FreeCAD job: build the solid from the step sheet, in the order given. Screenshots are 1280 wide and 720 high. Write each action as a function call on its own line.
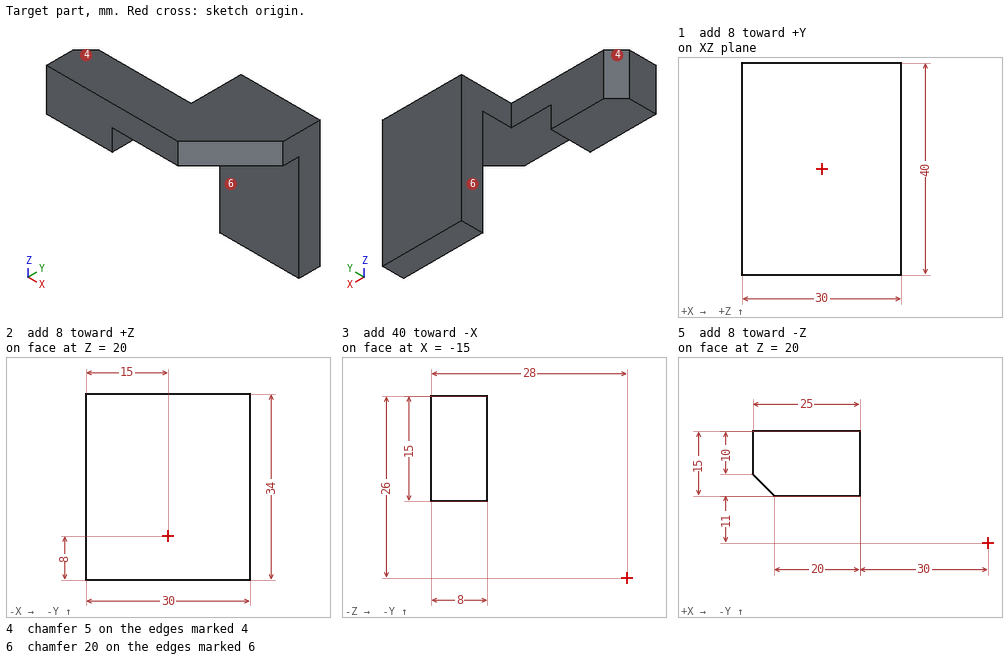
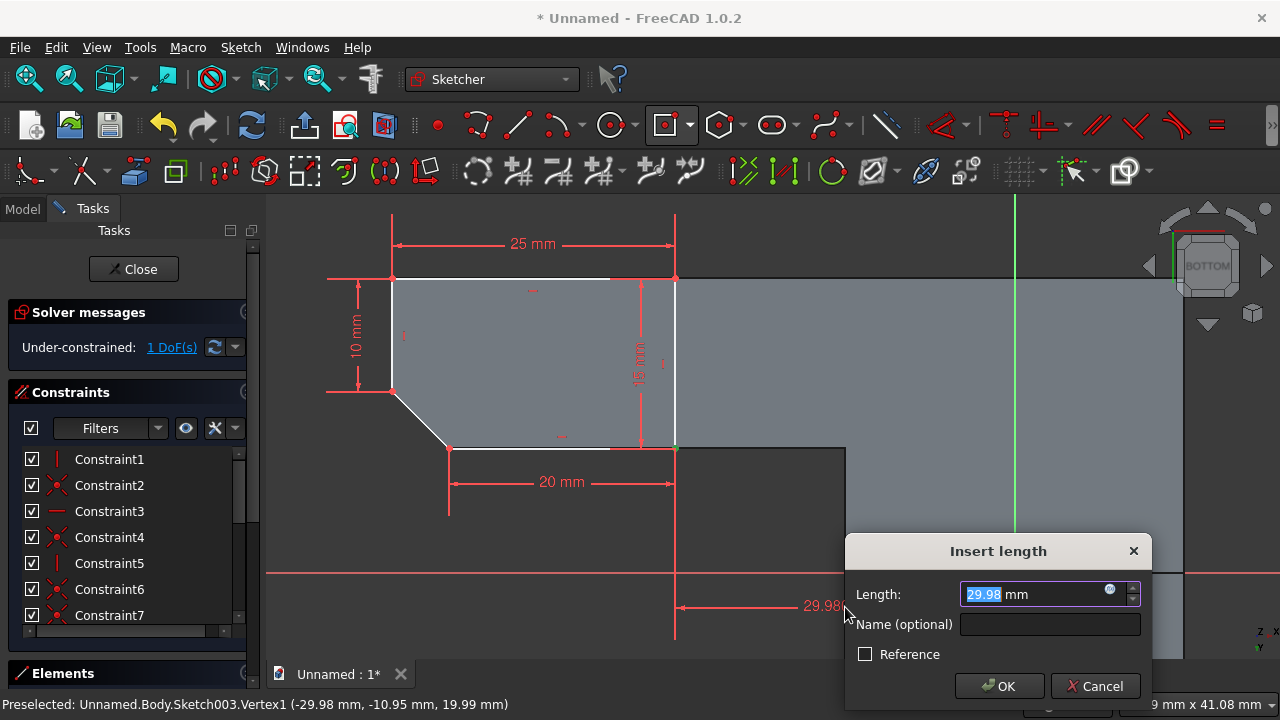
text(30)
key(Return)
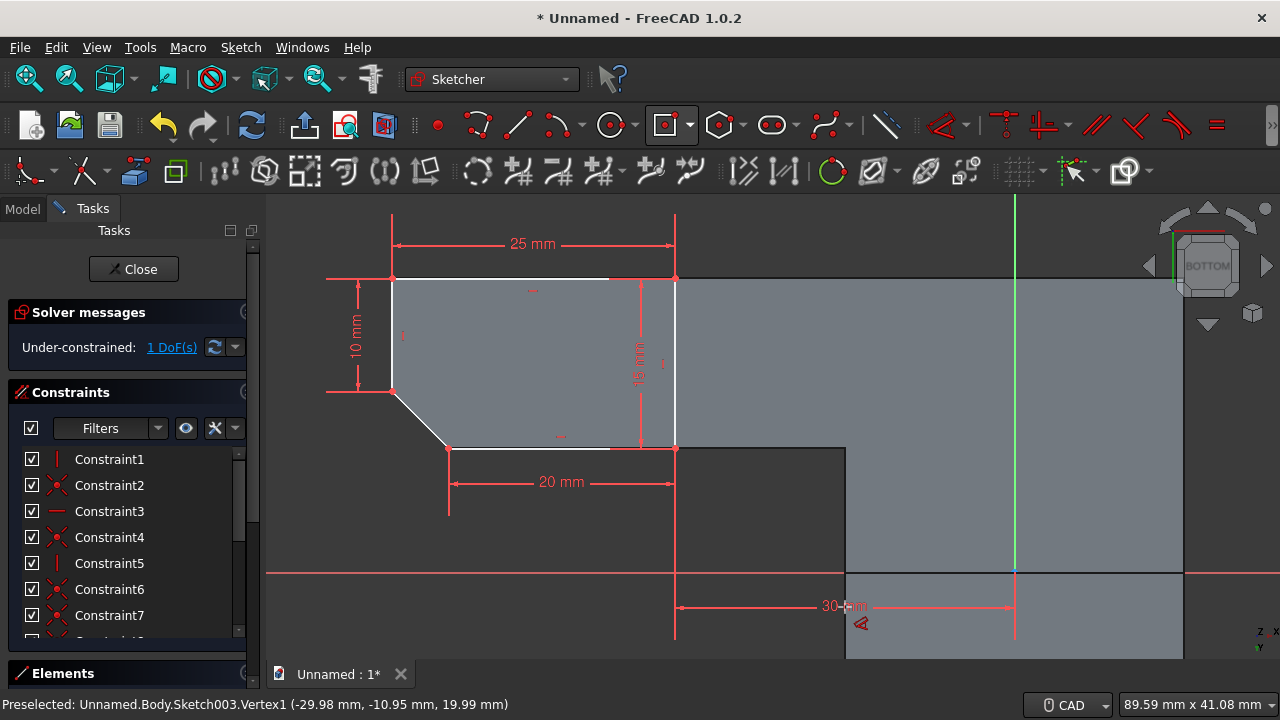
click(675, 449)
click(1049, 511)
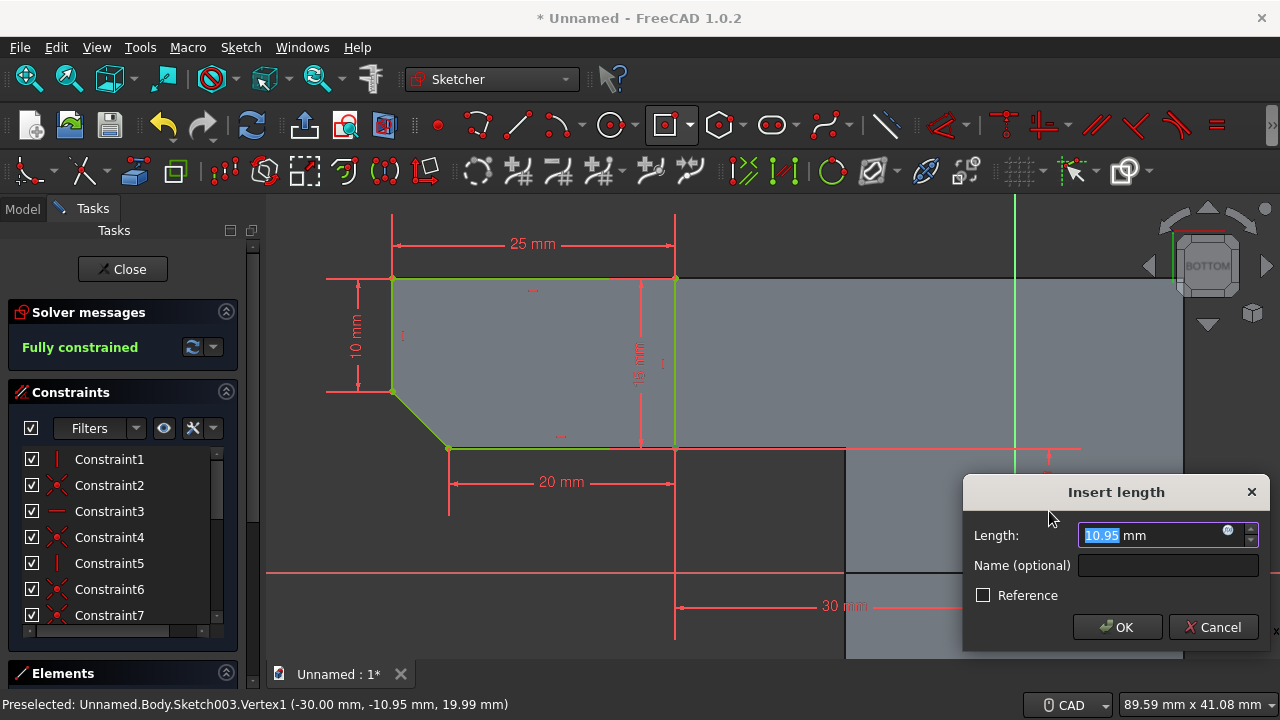
text(11)
key(Return)
key(Escape)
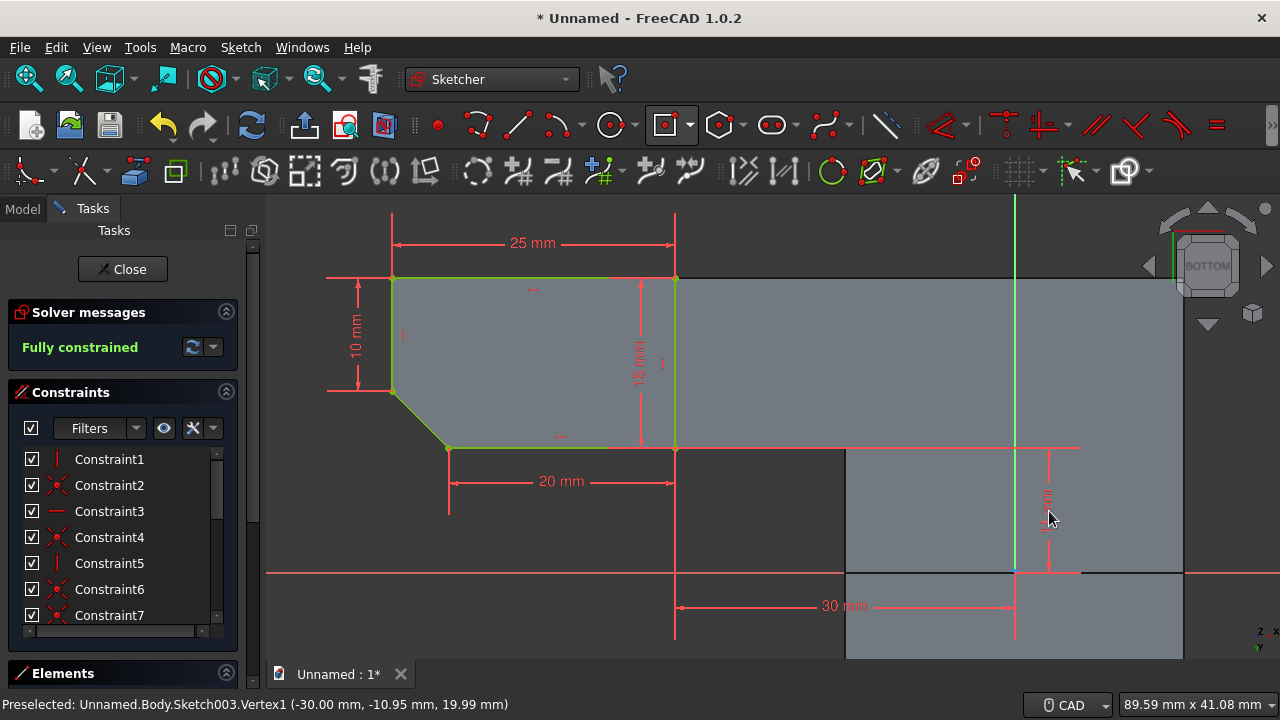
click(123, 269)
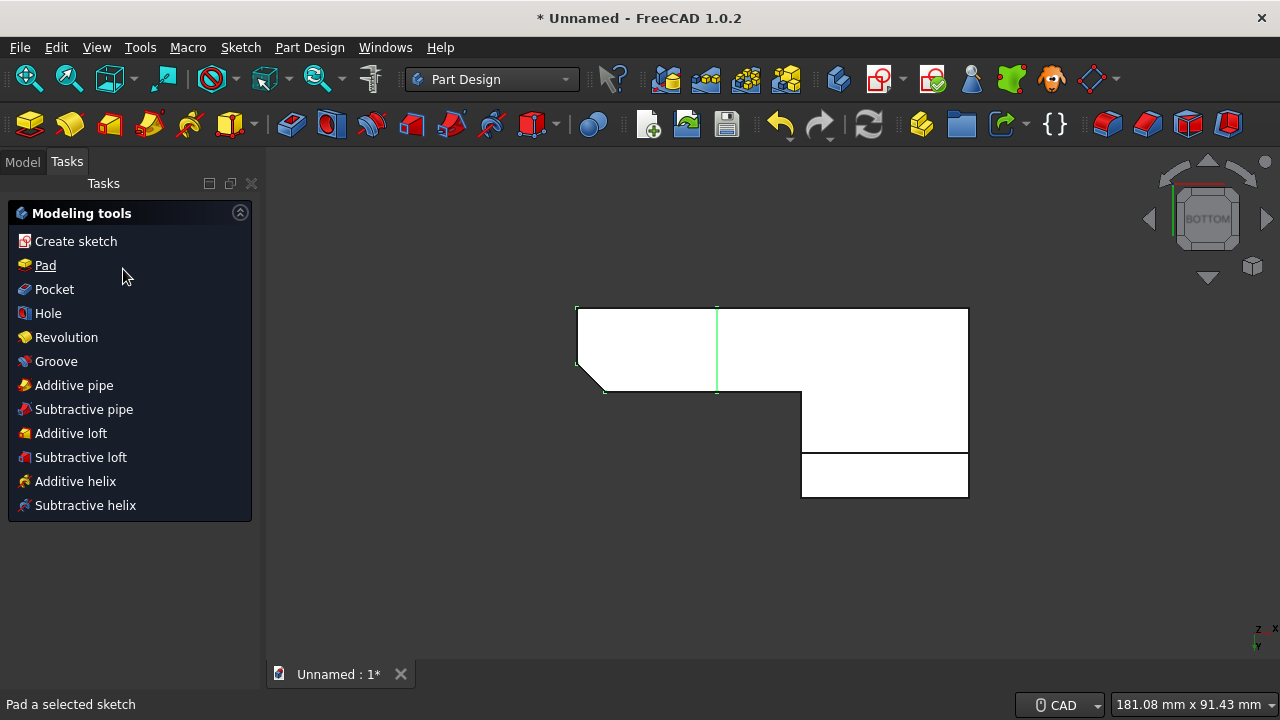
click(30, 124)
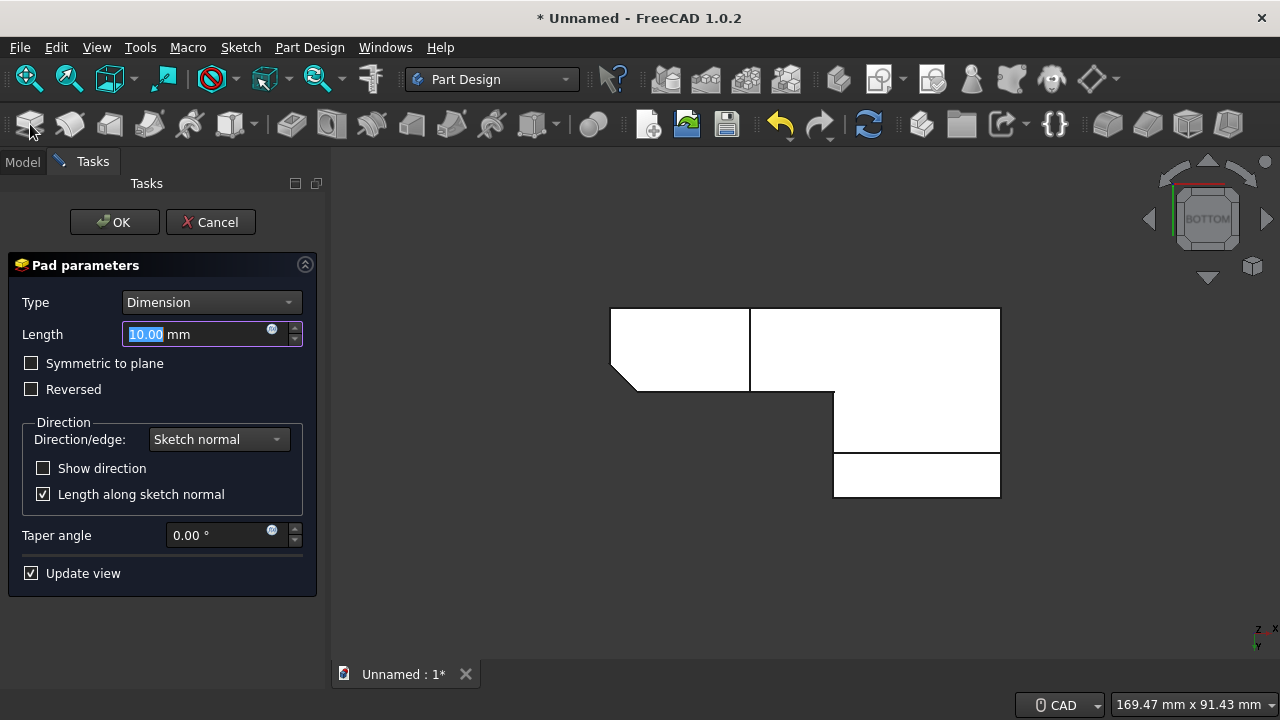
text(8)
key(Tab)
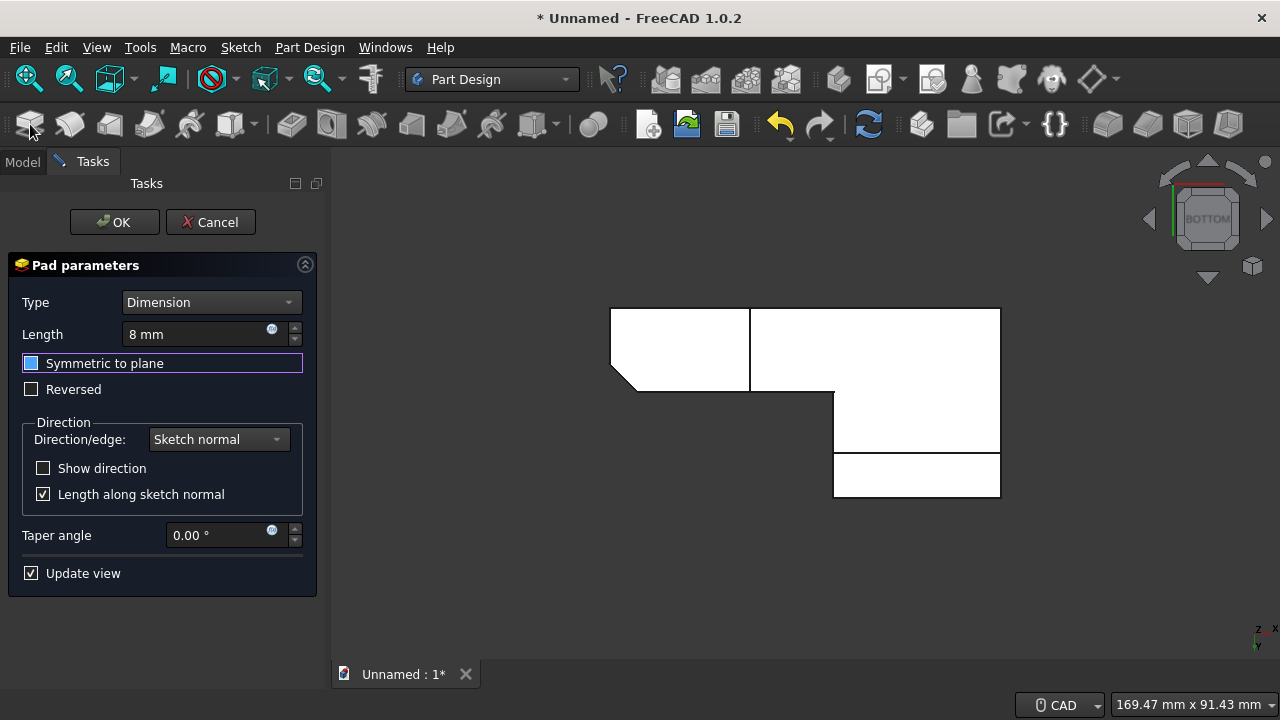
click(115, 222)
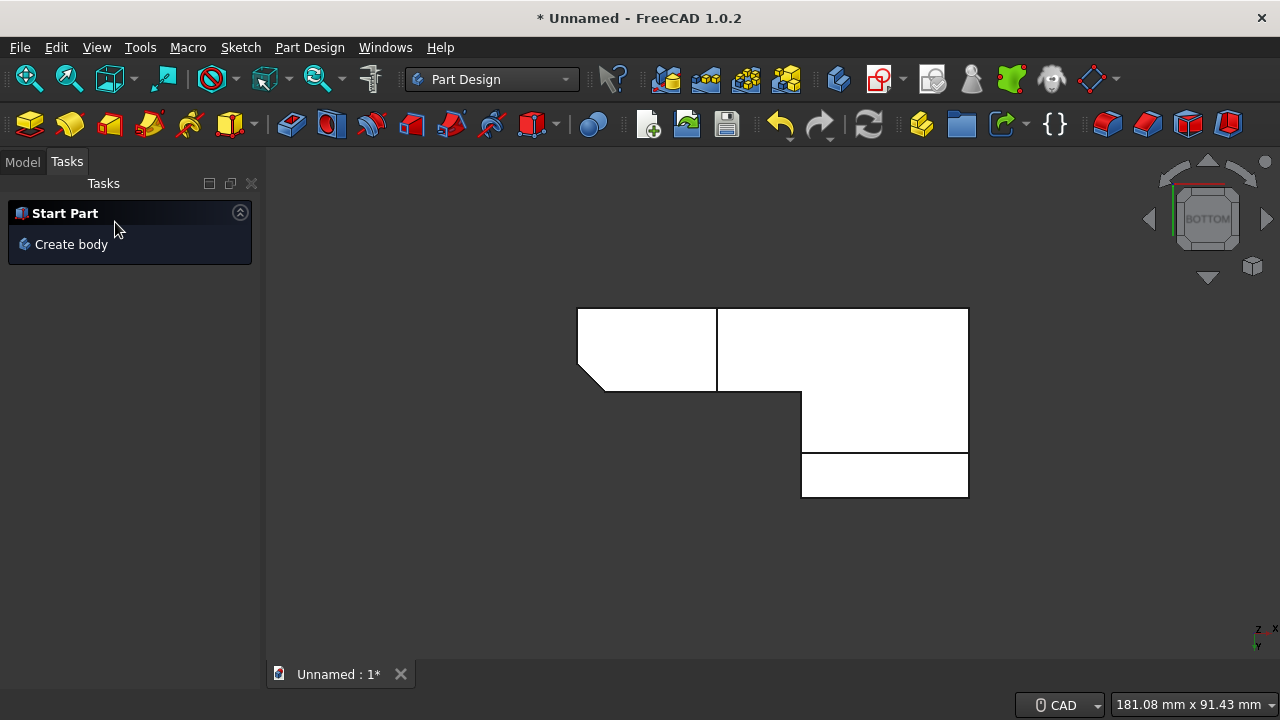
click(30, 80)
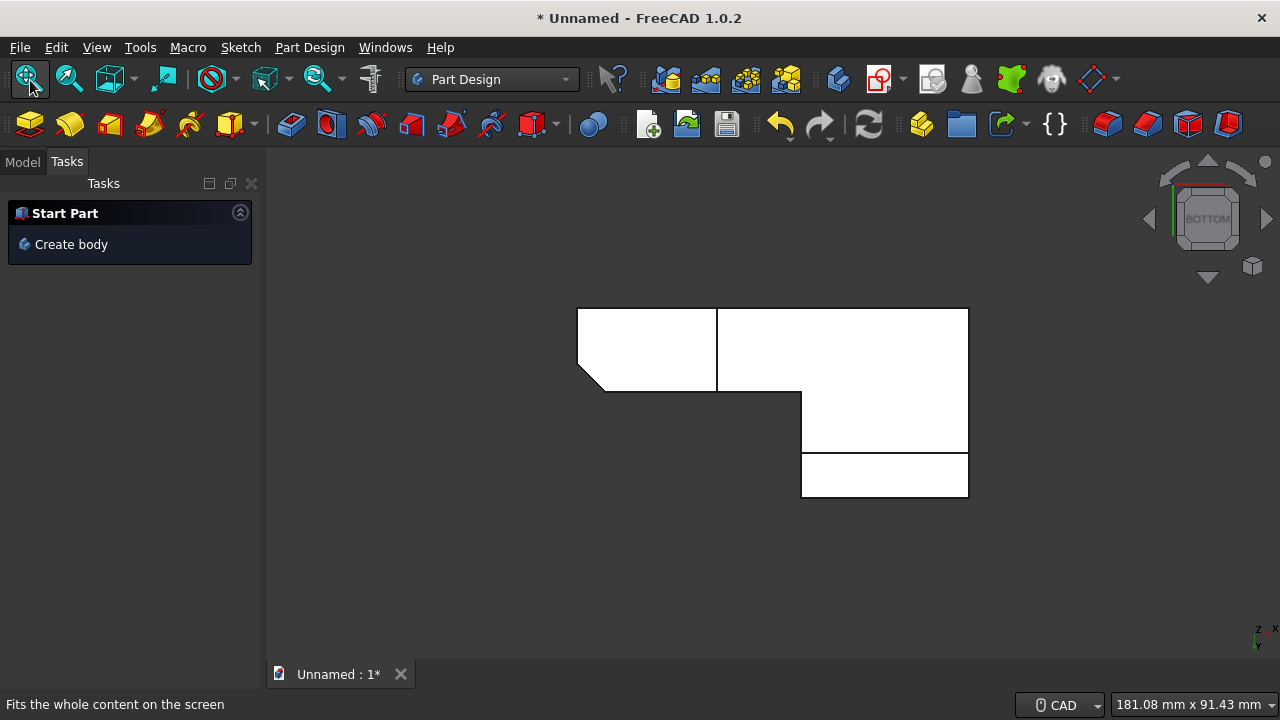
key(0)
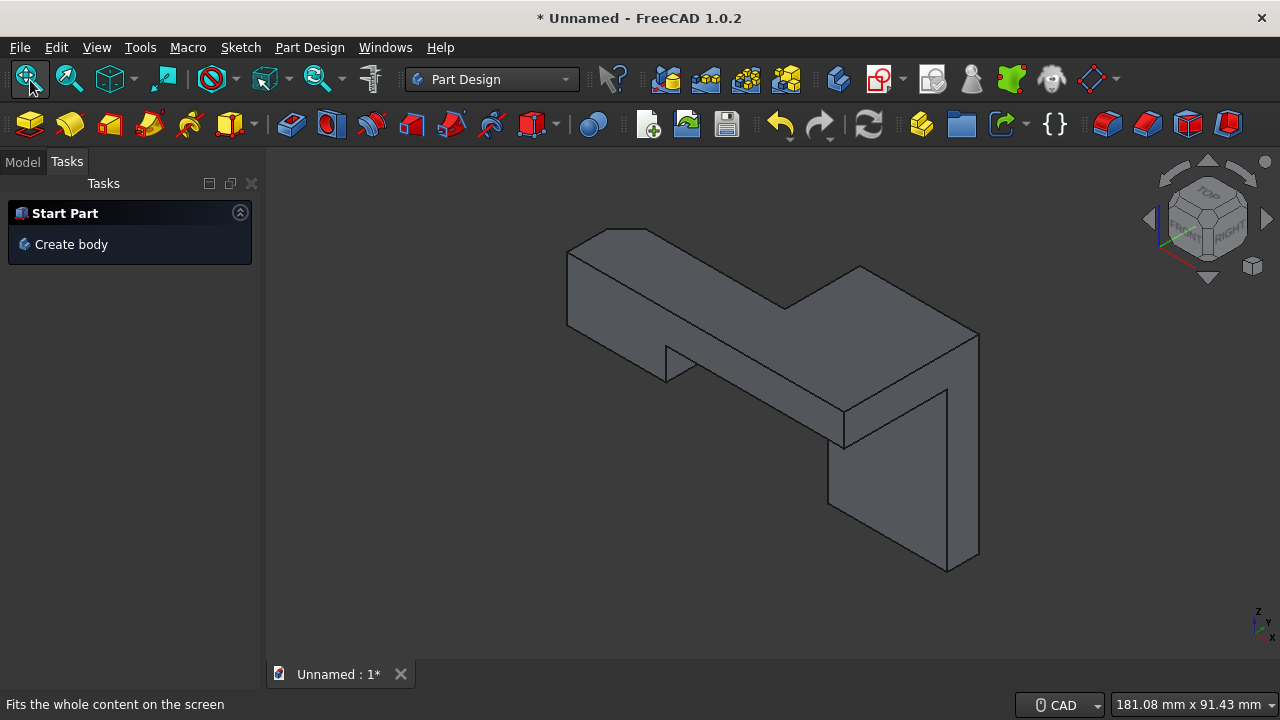
click(844, 429)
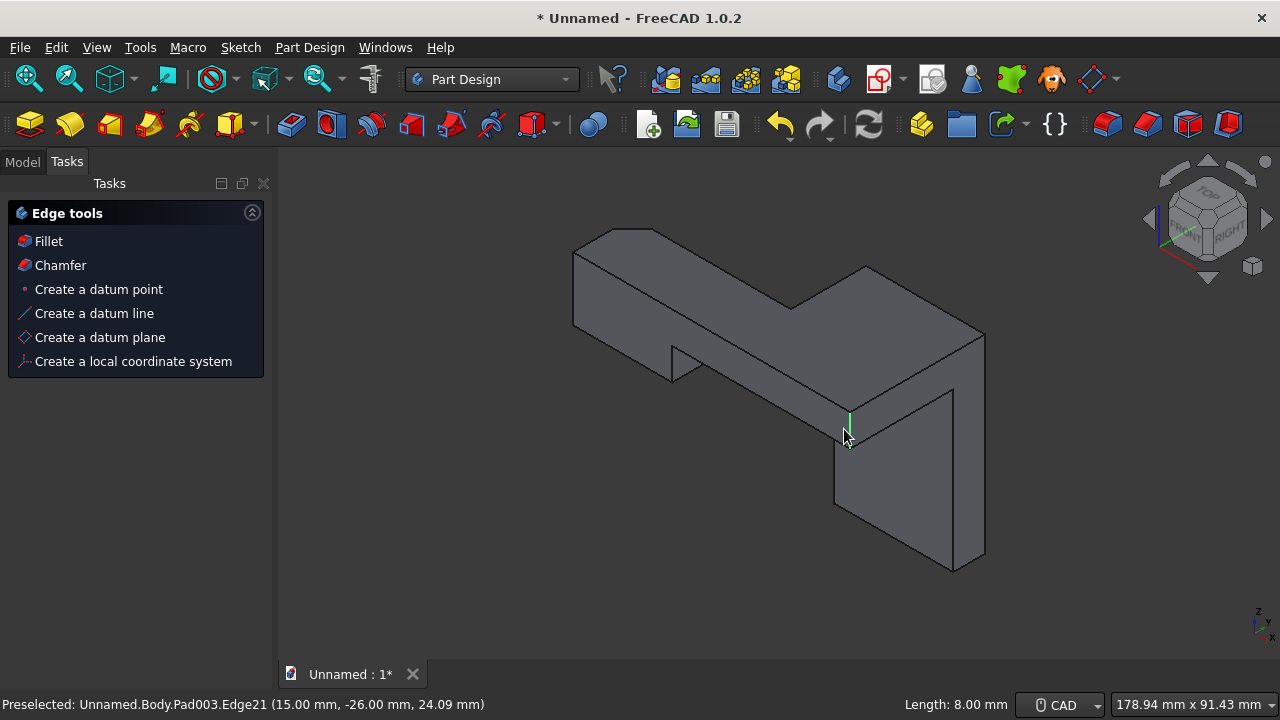
click(1148, 124)